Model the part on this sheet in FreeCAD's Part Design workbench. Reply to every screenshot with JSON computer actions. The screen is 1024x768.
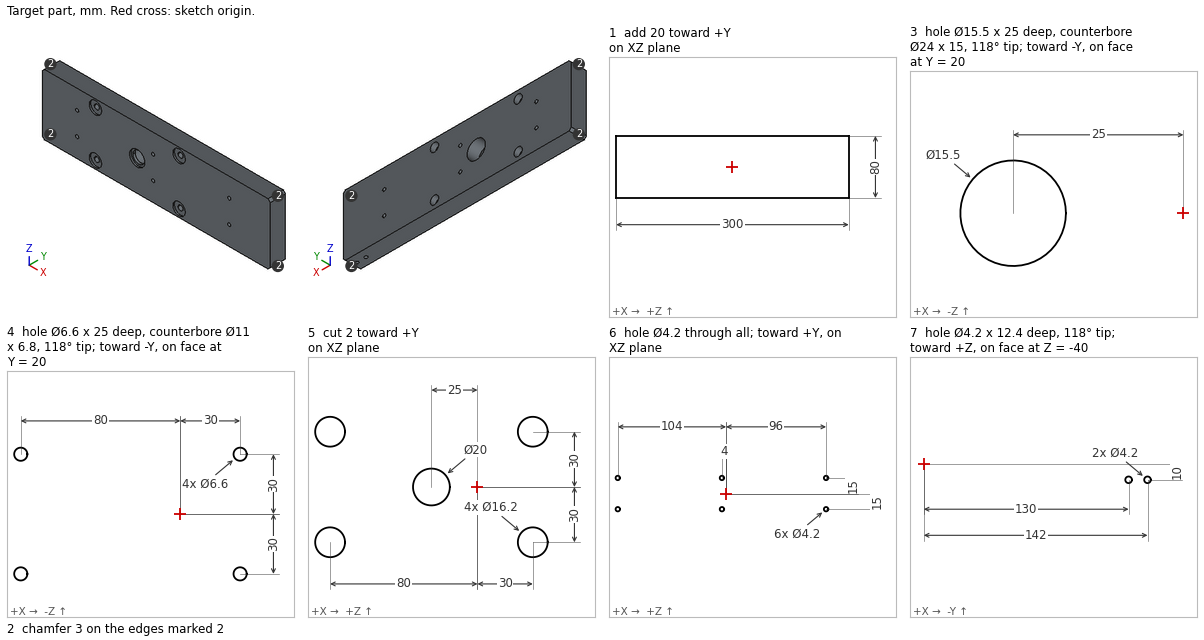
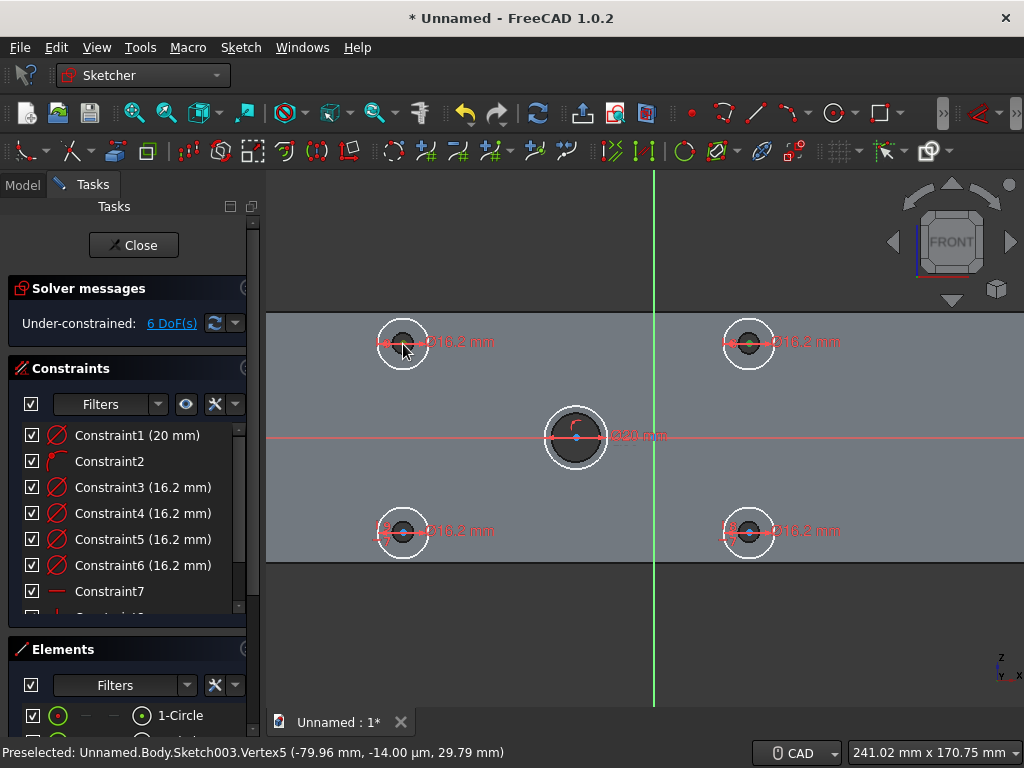
{"action": "key", "text": "h"}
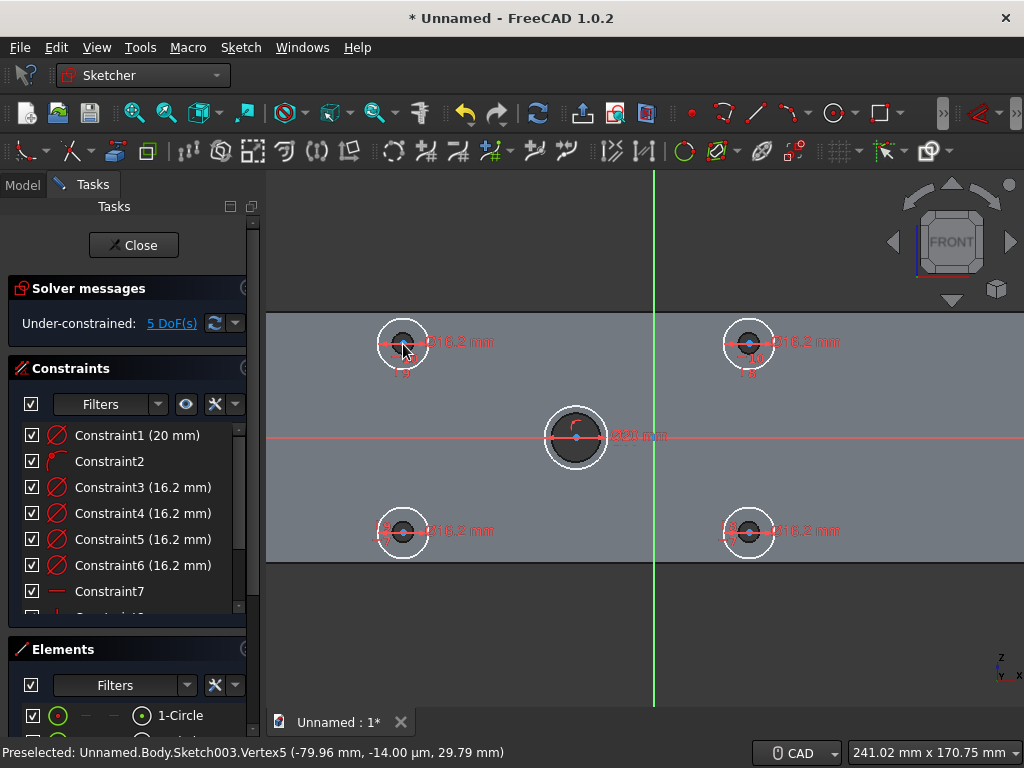
{"action": "left_click", "coordinate": [978, 114]}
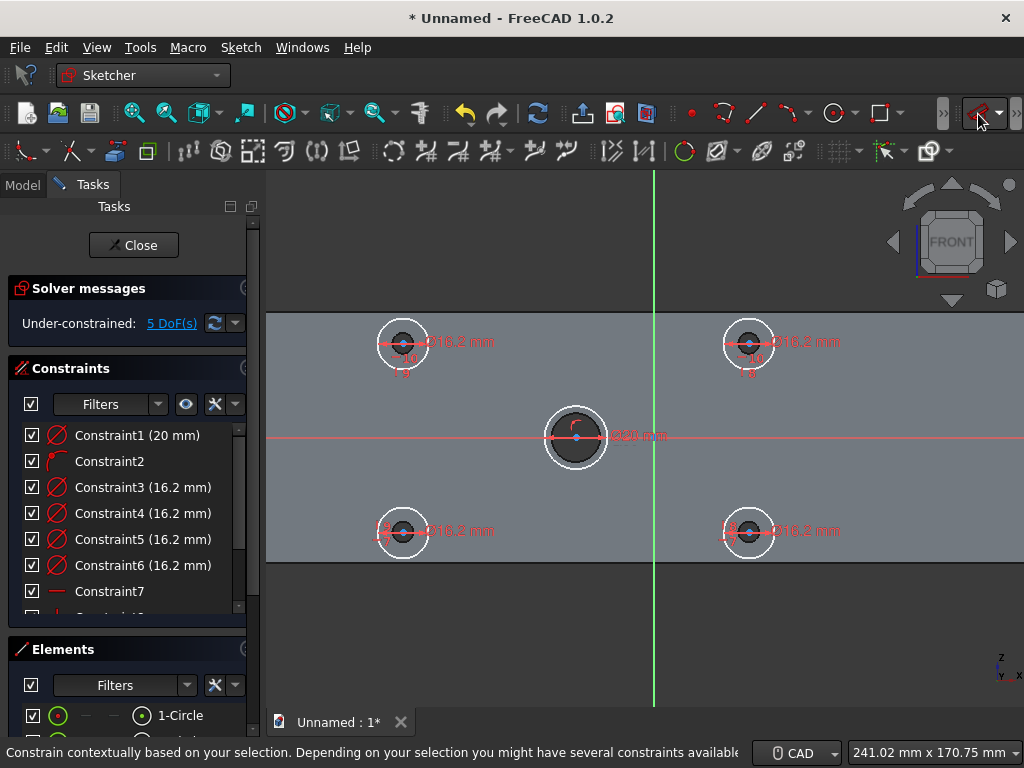
{"action": "left_click", "coordinate": [576, 438]}
{"action": "left_click", "coordinate": [615, 472]}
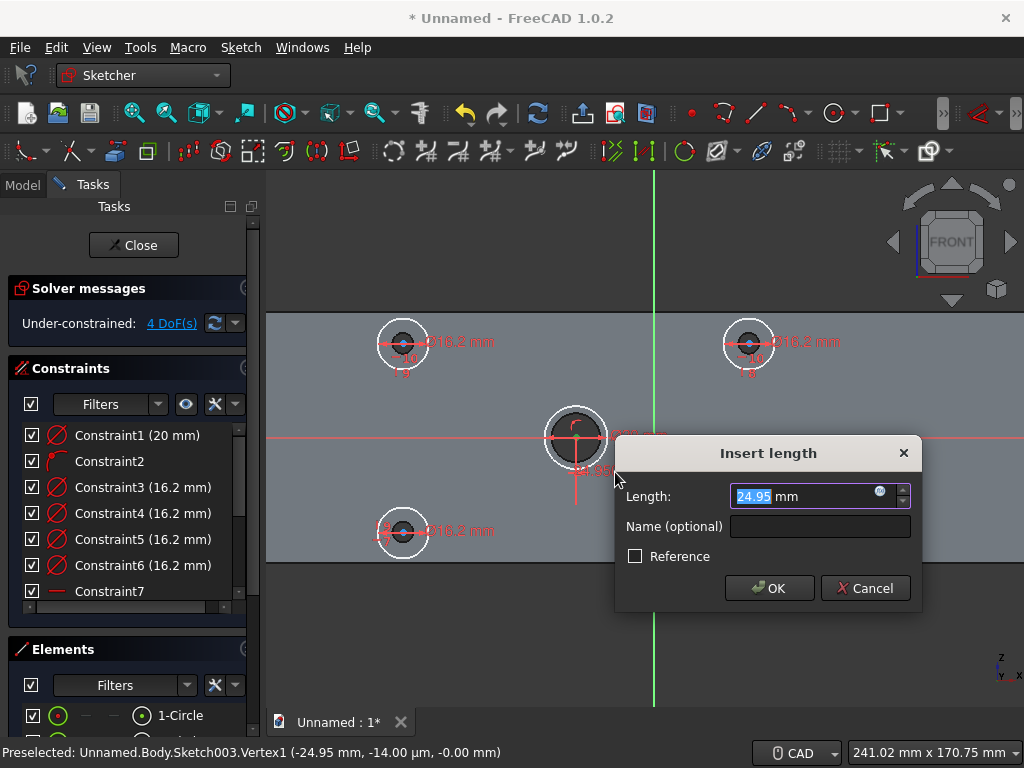
{"action": "type", "text": "25"}
{"action": "key", "text": "Return"}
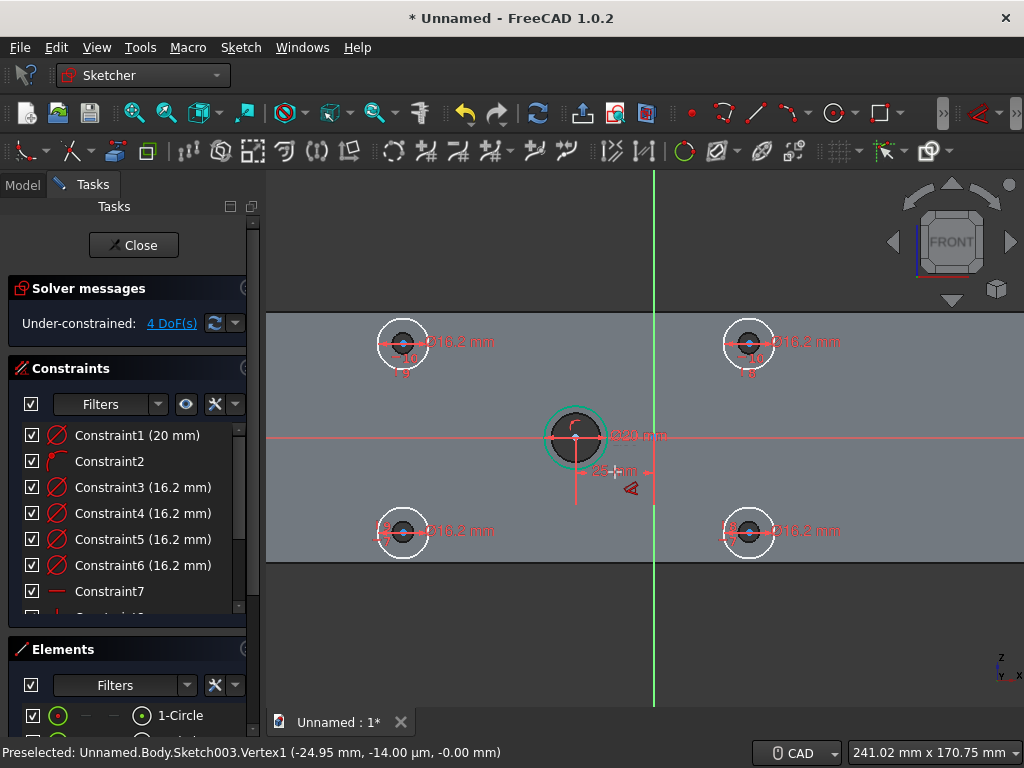
{"action": "left_click", "coordinate": [749, 533]}
{"action": "left_click", "coordinate": [702, 567]}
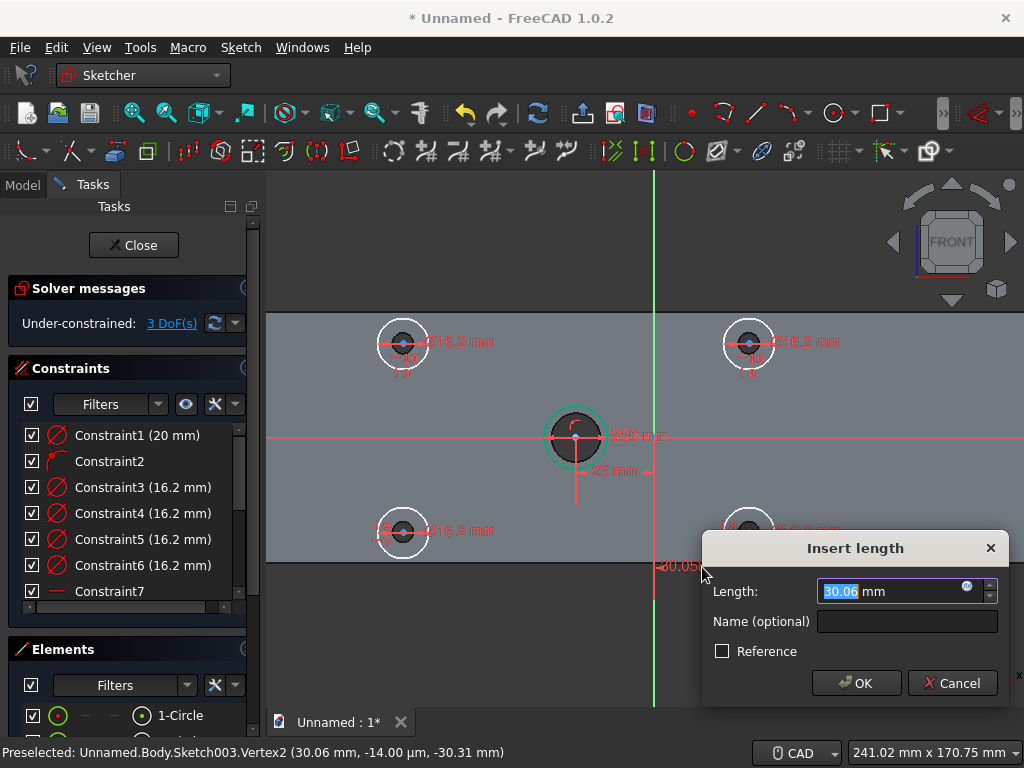
{"action": "type", "text": "30"}
{"action": "key", "text": "Return"}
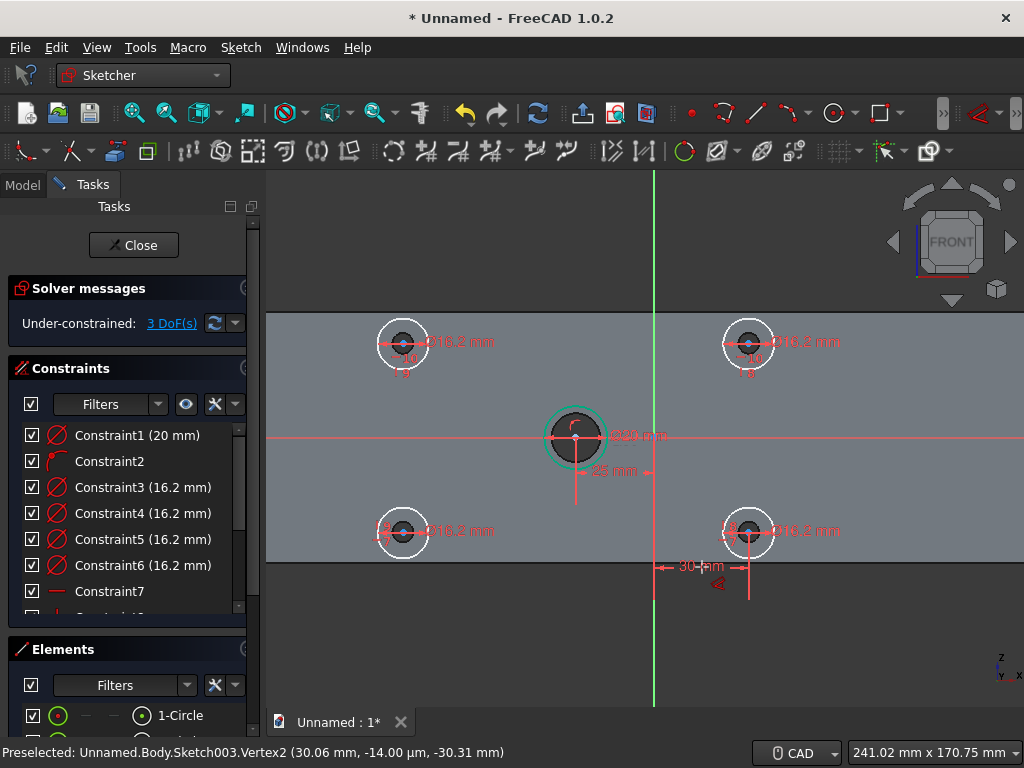
{"action": "left_click", "coordinate": [749, 533]}
{"action": "left_click", "coordinate": [783, 485]}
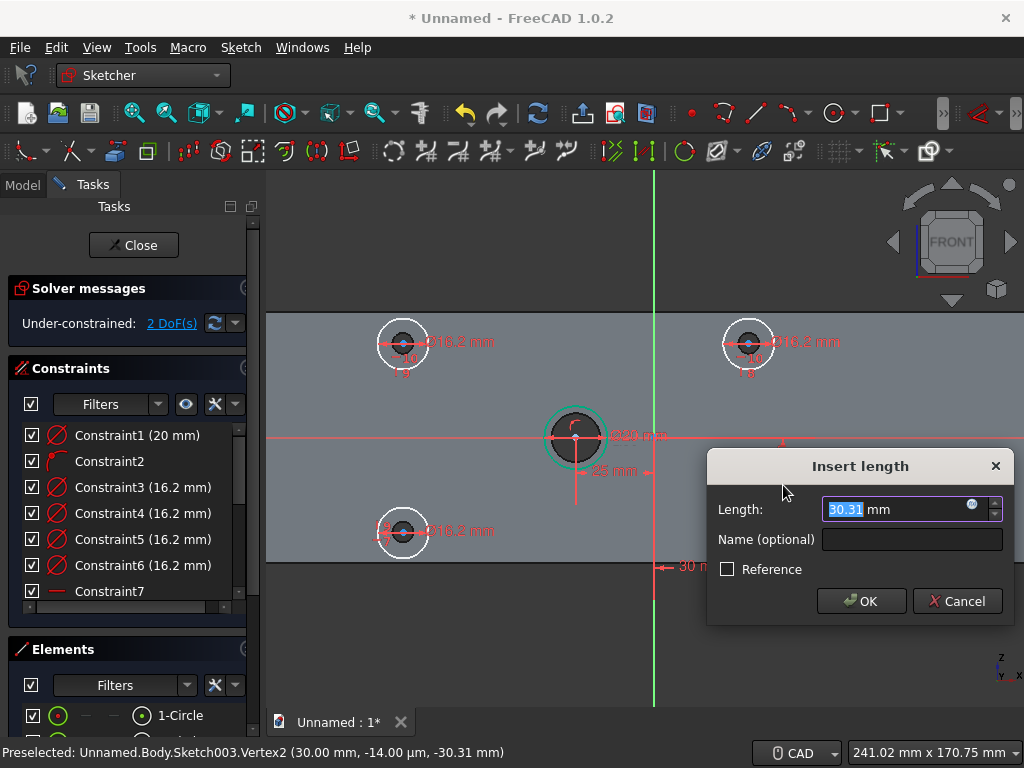
{"action": "type", "text": "30"}
{"action": "key", "text": "Return"}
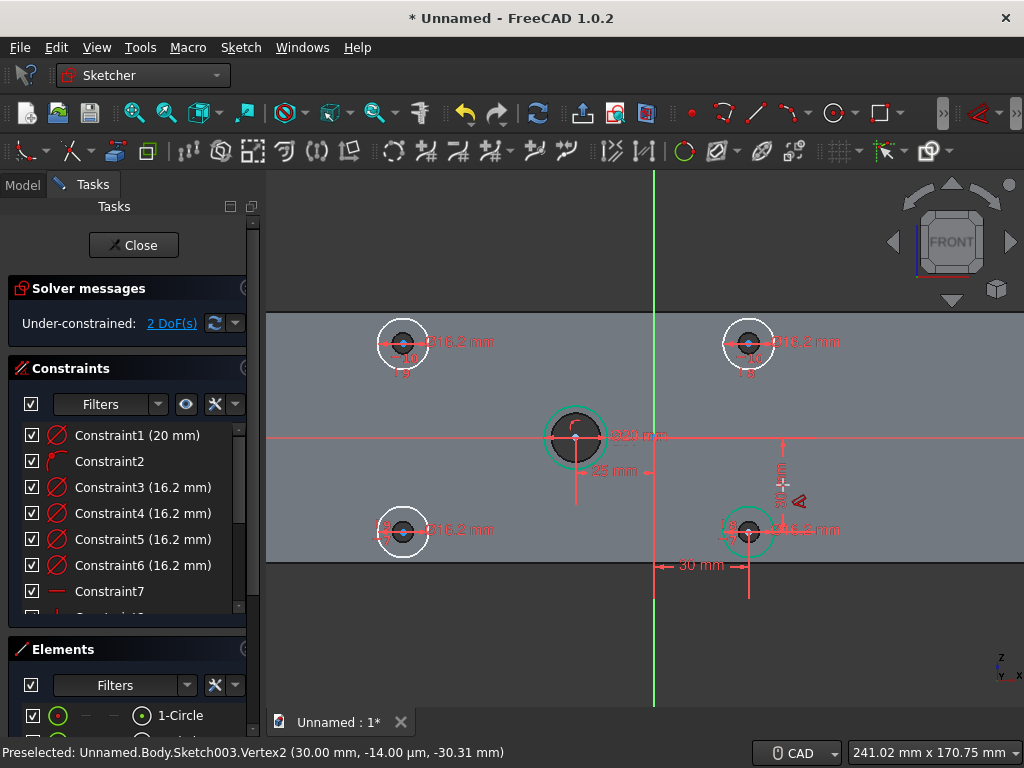
{"action": "left_click", "coordinate": [403, 532]}
{"action": "left_click", "coordinate": [529, 566]}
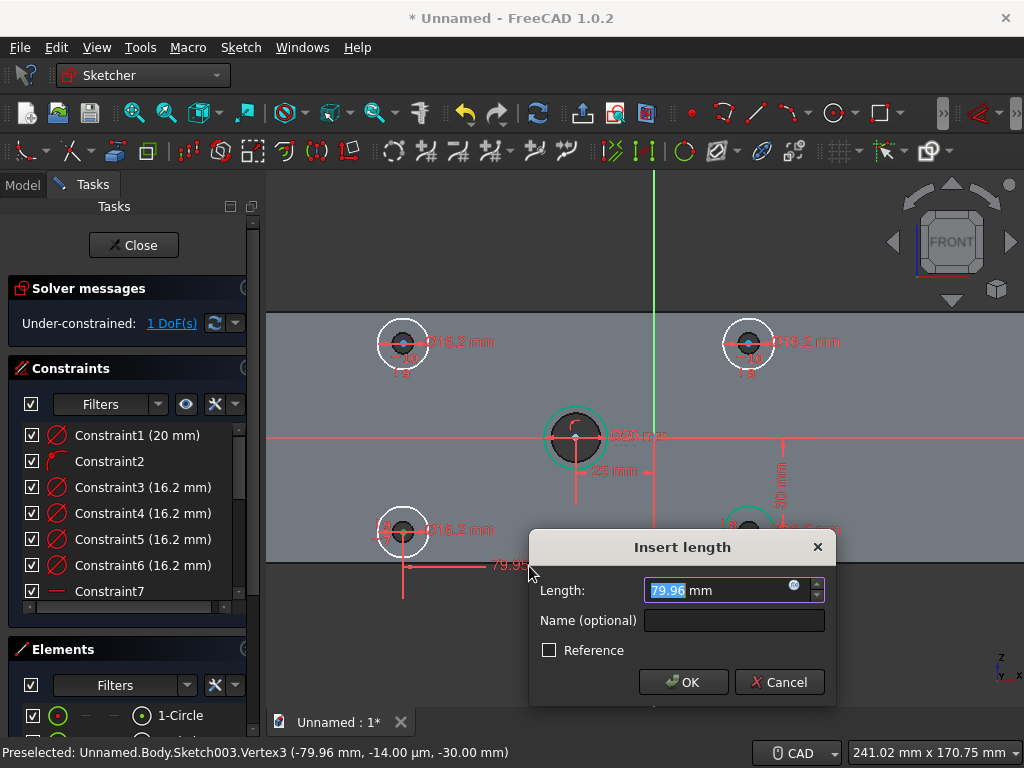
{"action": "type", "text": "80"}
{"action": "key", "text": "Return"}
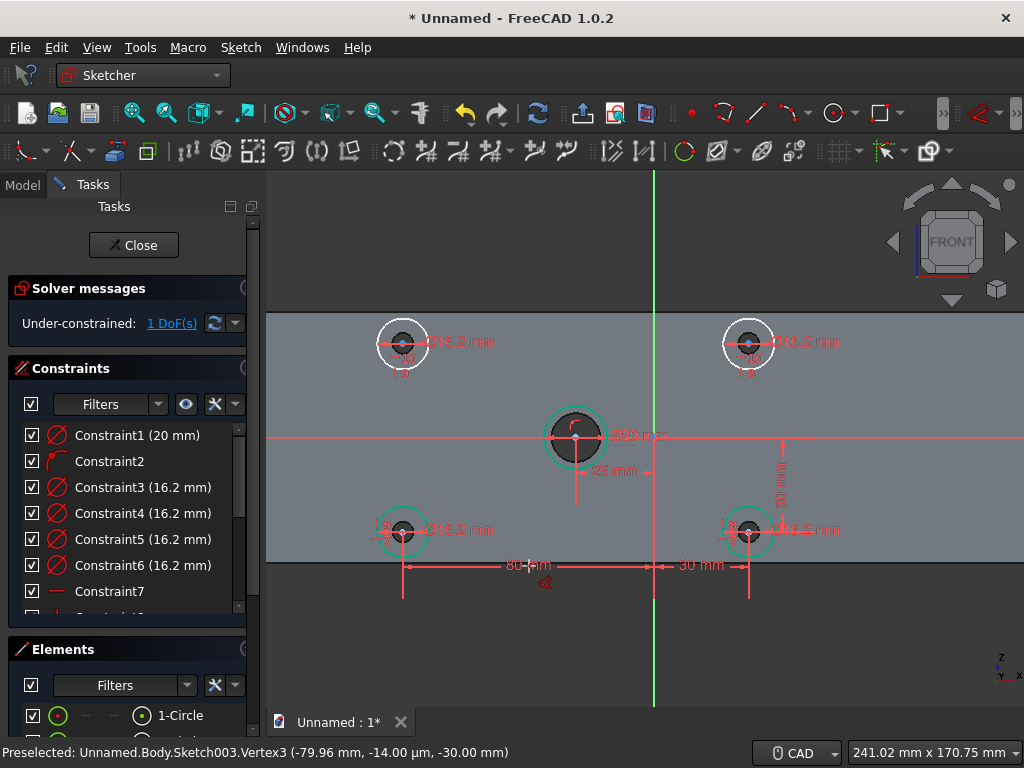
{"action": "left_click", "coordinate": [749, 344]}
{"action": "left_click", "coordinate": [783, 391]}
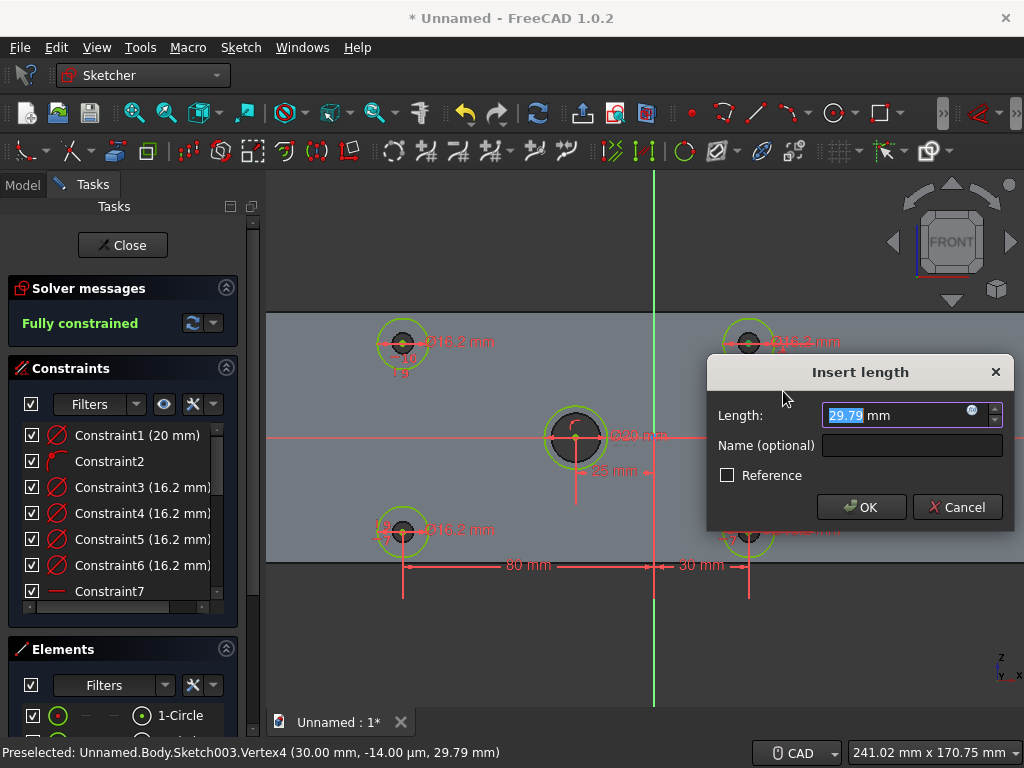
{"action": "type", "text": "30"}
{"action": "key", "text": "Return"}
{"action": "key", "text": "Escape"}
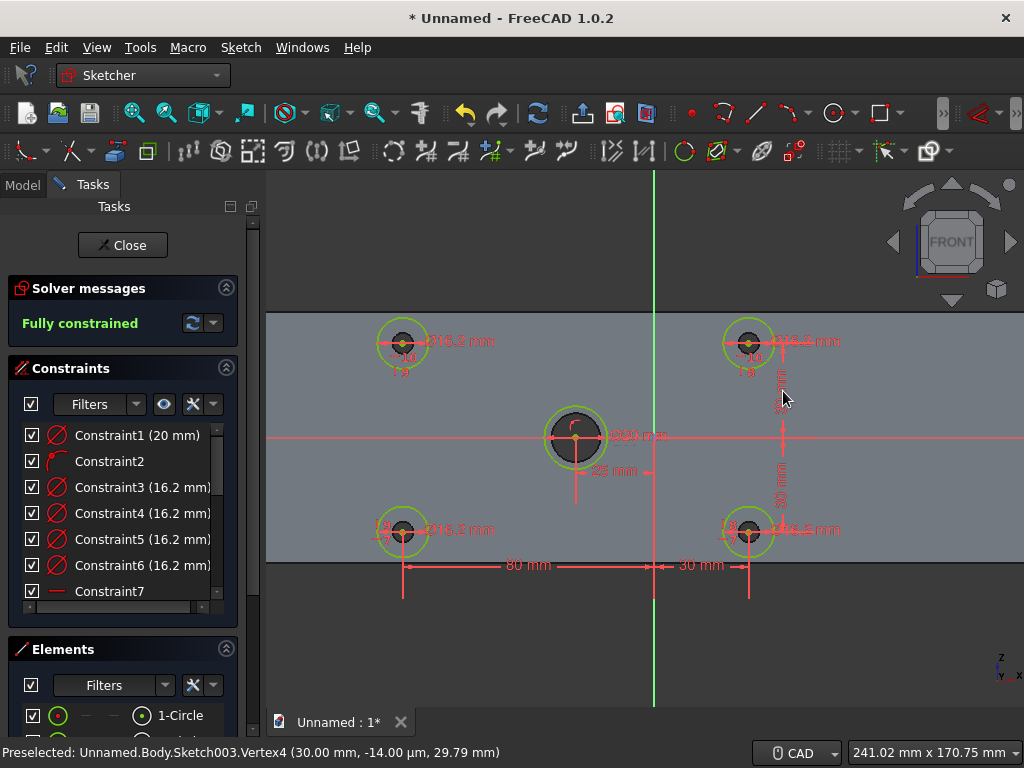
{"action": "left_click", "coordinate": [123, 245]}